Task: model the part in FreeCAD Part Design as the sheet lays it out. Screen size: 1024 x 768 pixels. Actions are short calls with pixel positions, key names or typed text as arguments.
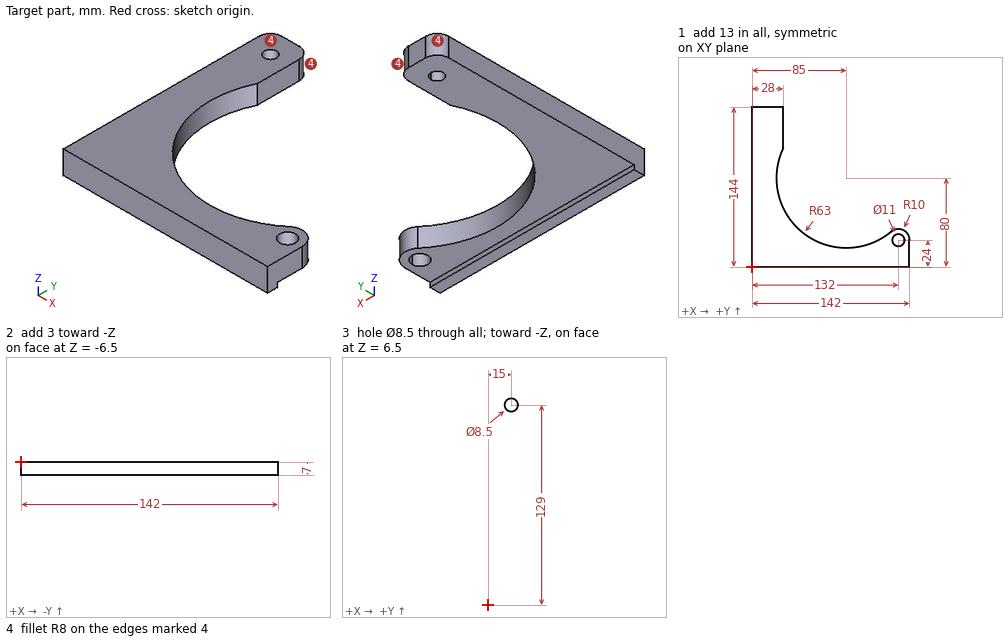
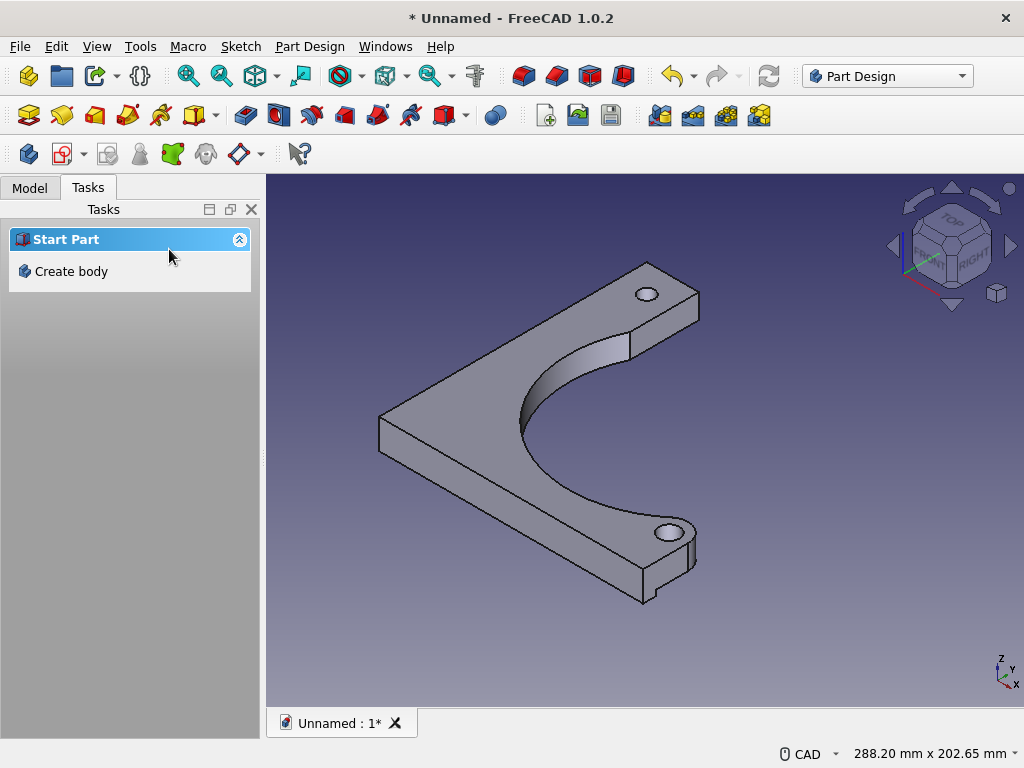
key(1)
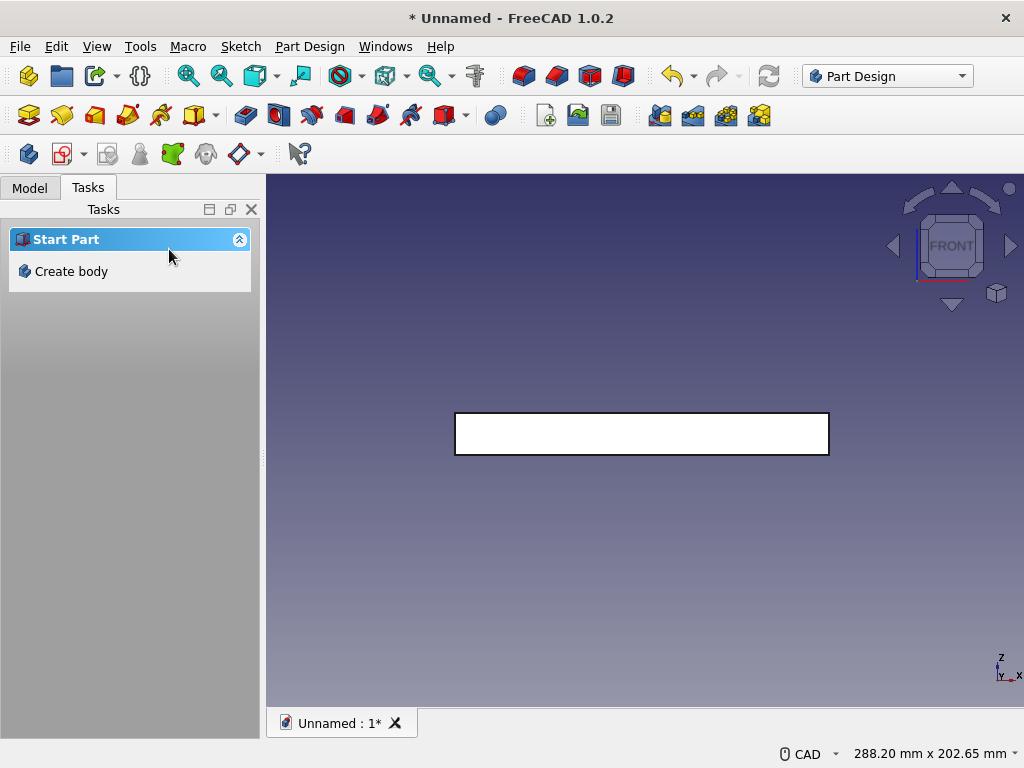
key(3)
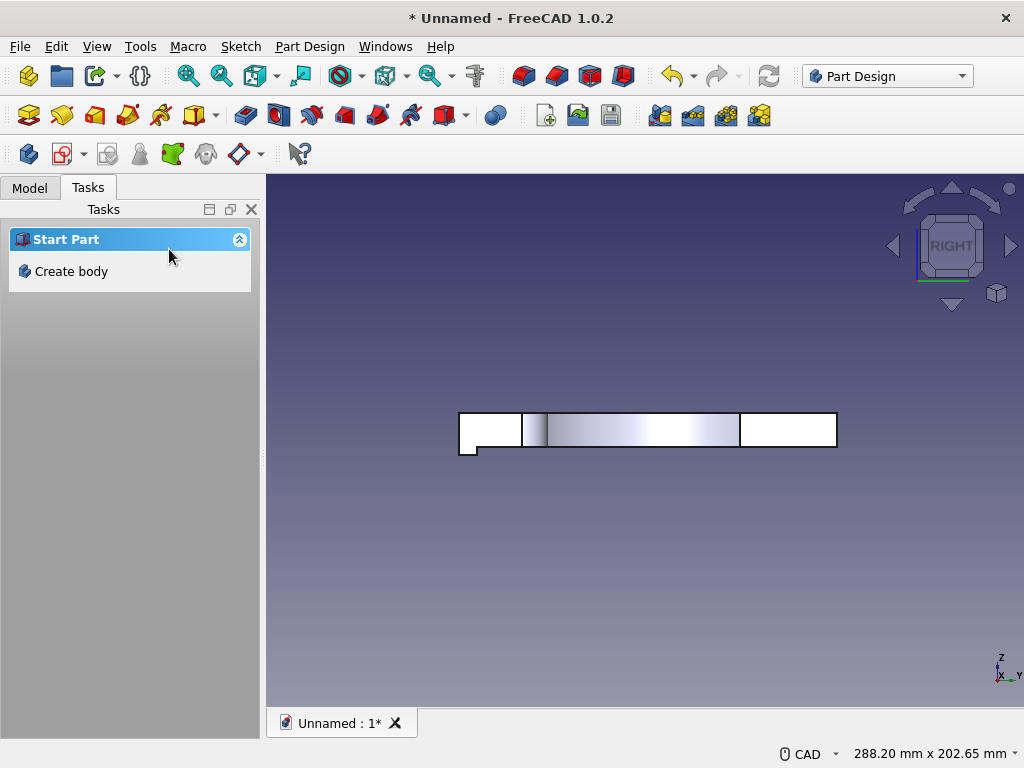
click(837, 429)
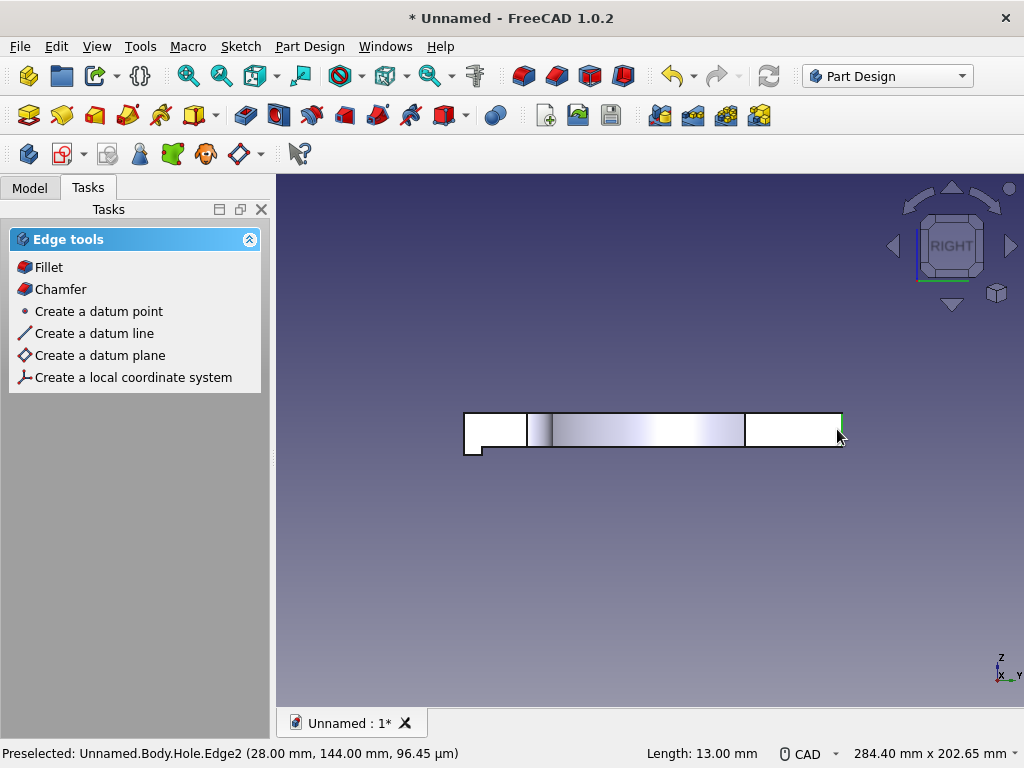
key(5)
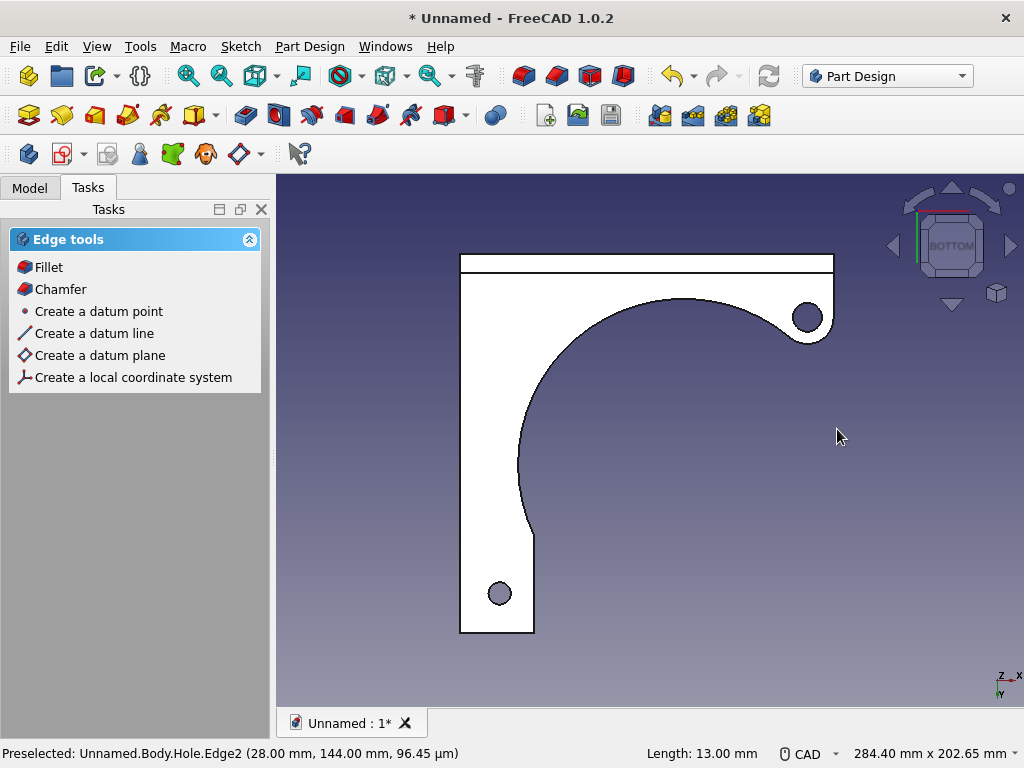
key(4)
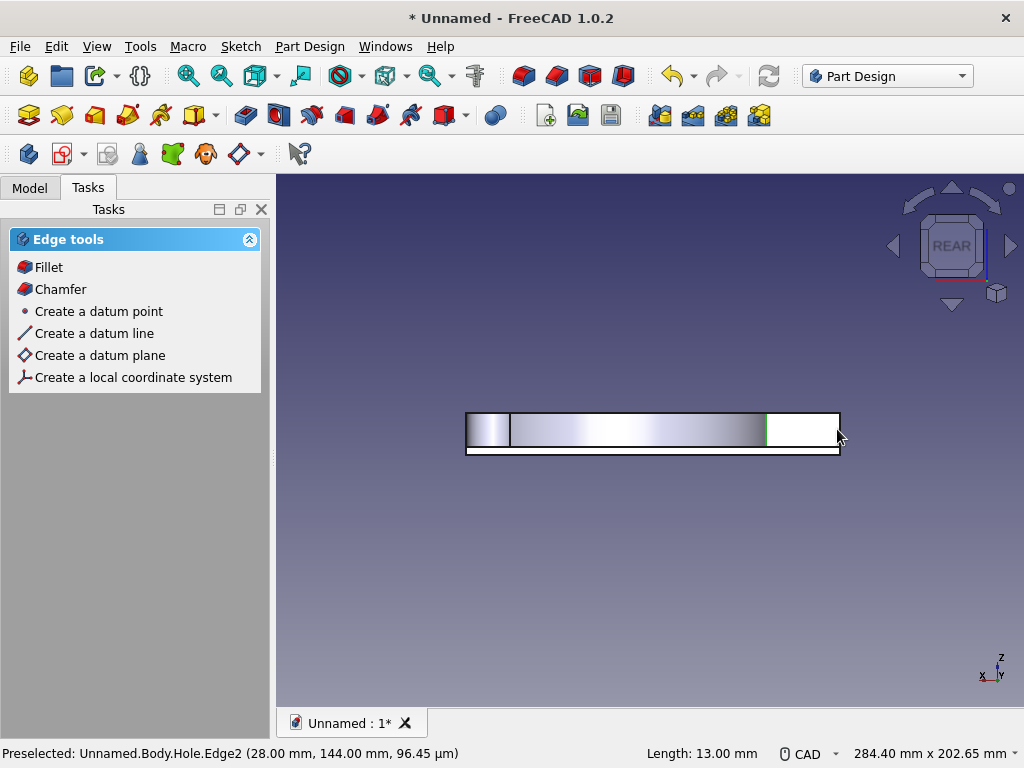
click(840, 429, ctrl)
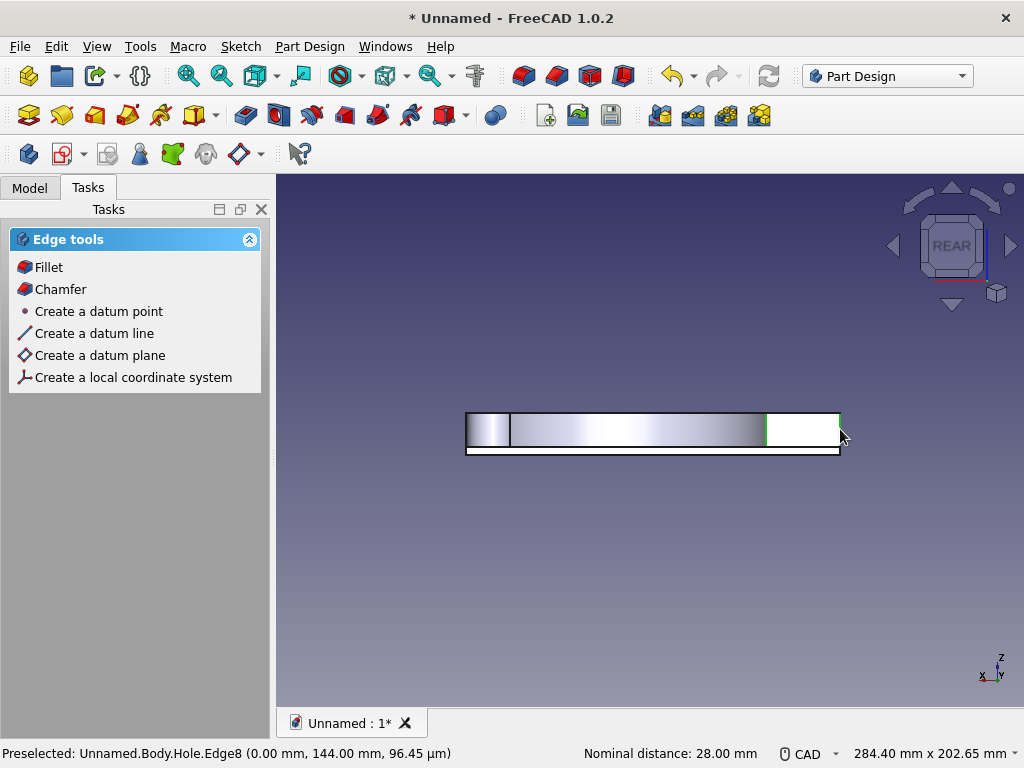
click(524, 76)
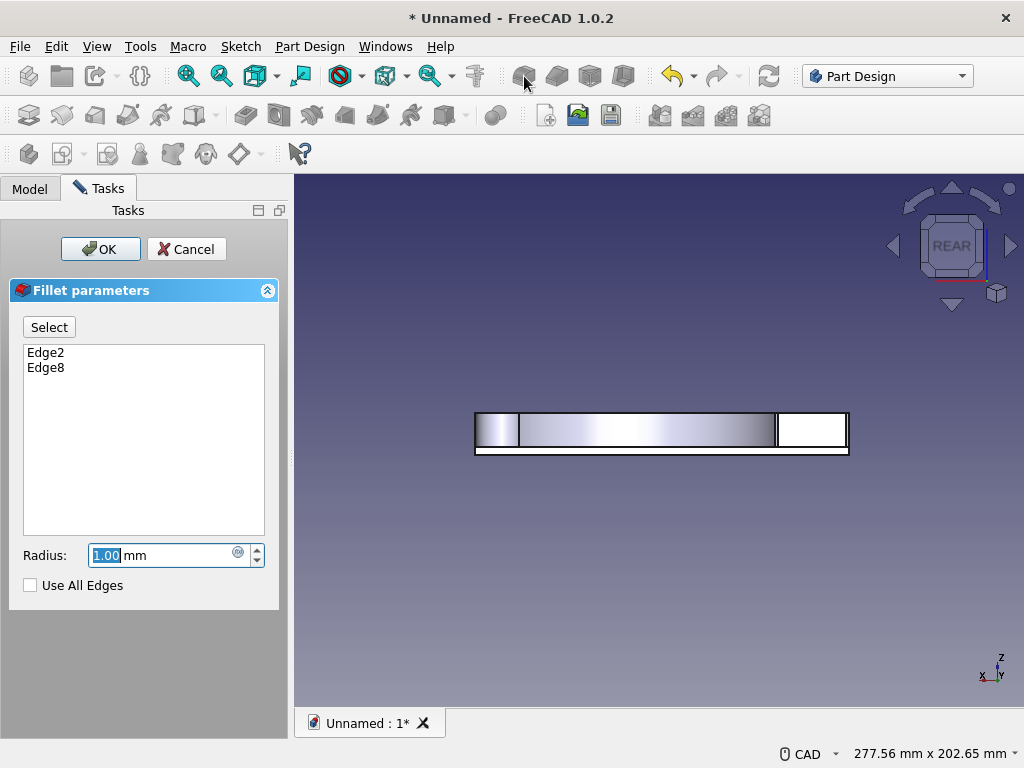
text(8)
key(Tab)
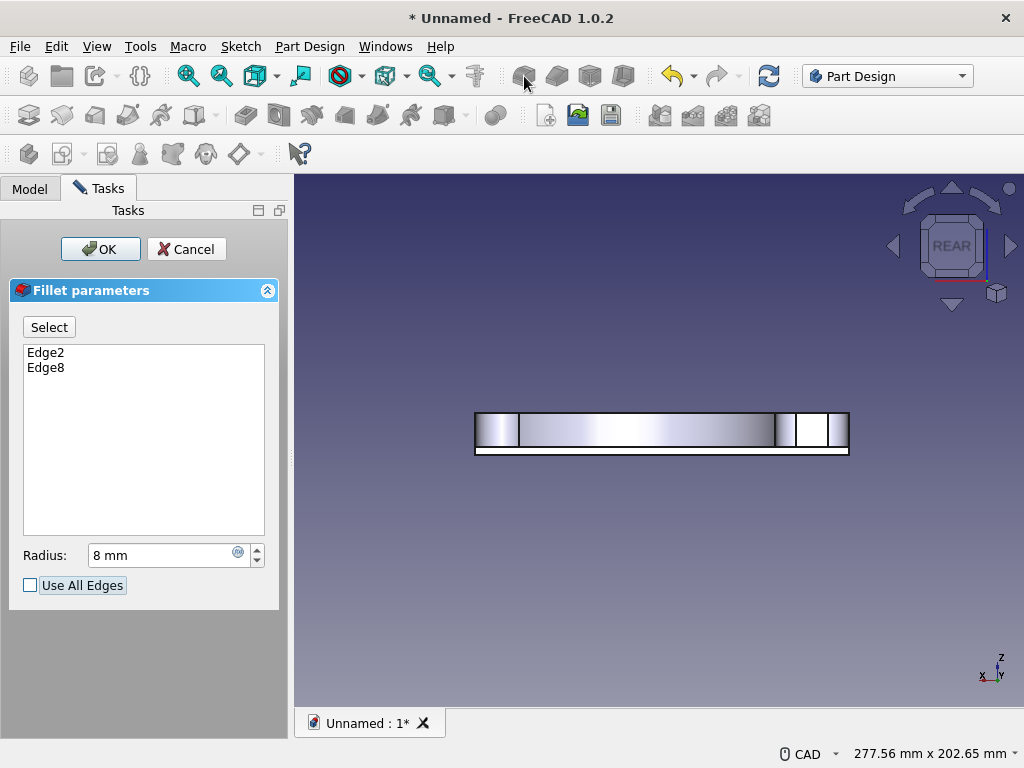
click(101, 249)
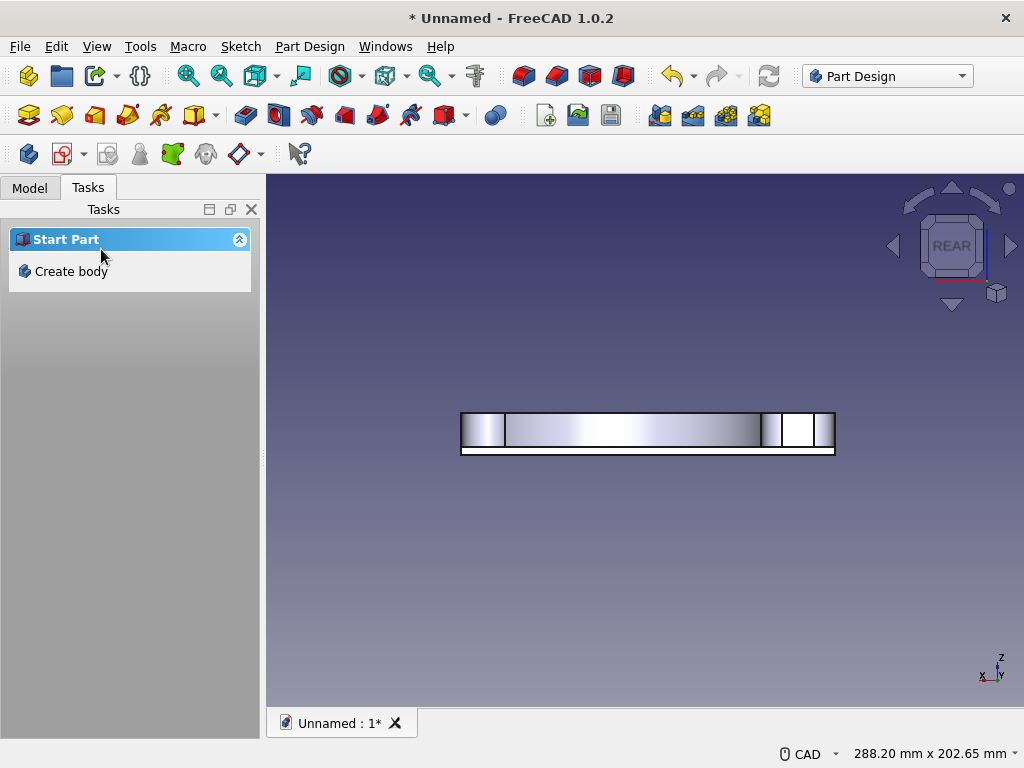
key(0)